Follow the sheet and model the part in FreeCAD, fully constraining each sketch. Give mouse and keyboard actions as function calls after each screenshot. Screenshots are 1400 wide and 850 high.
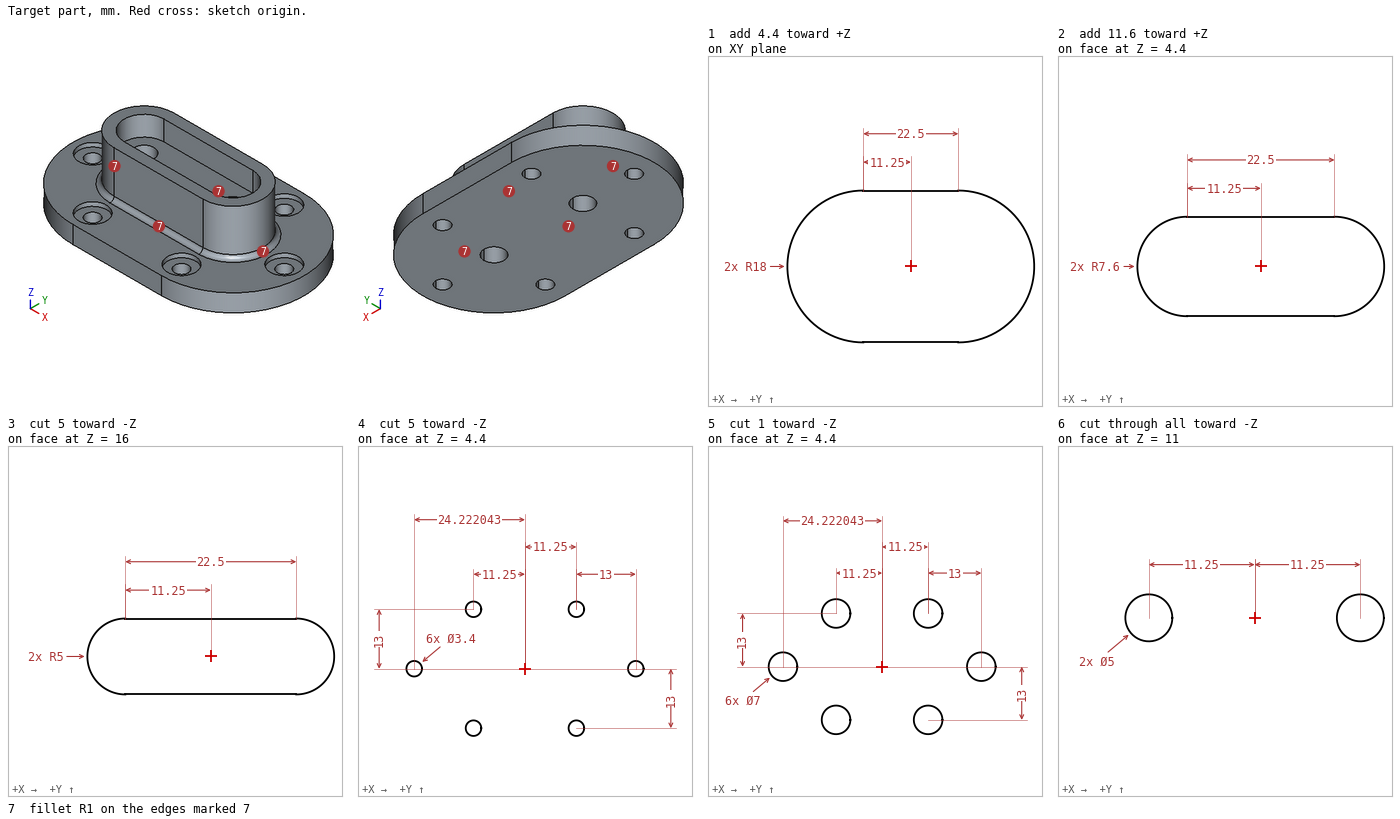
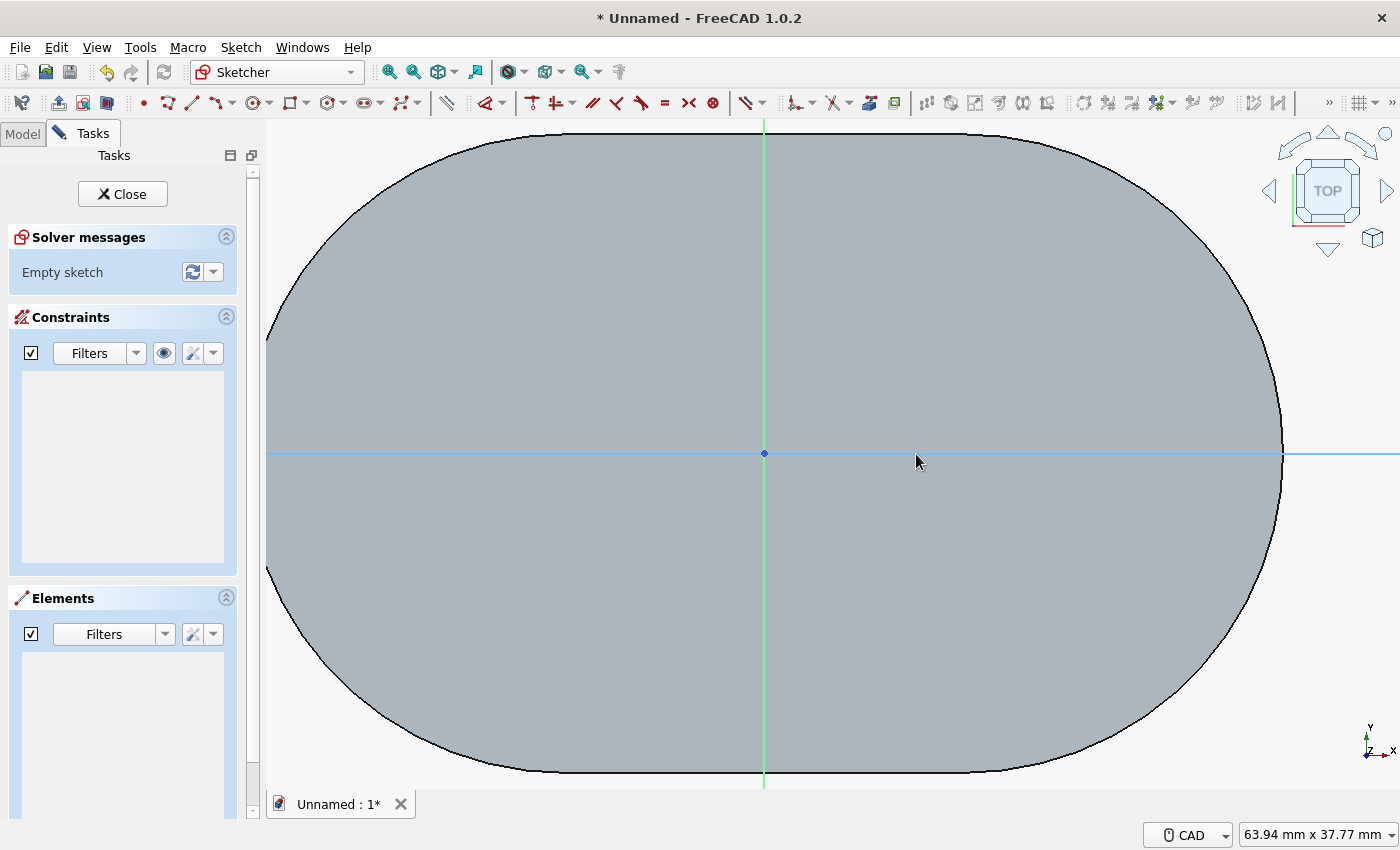
click(364, 104)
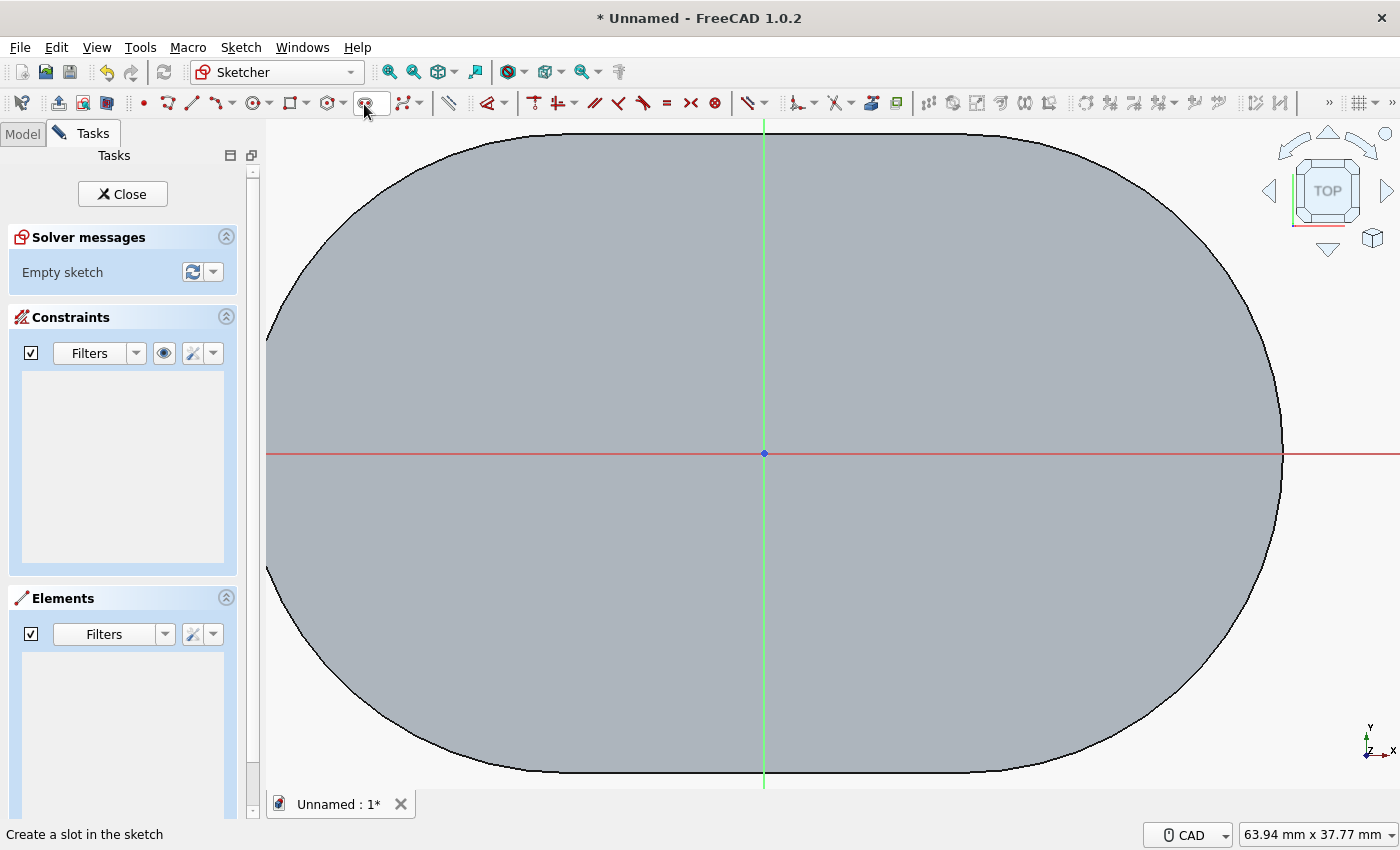
click(565, 454)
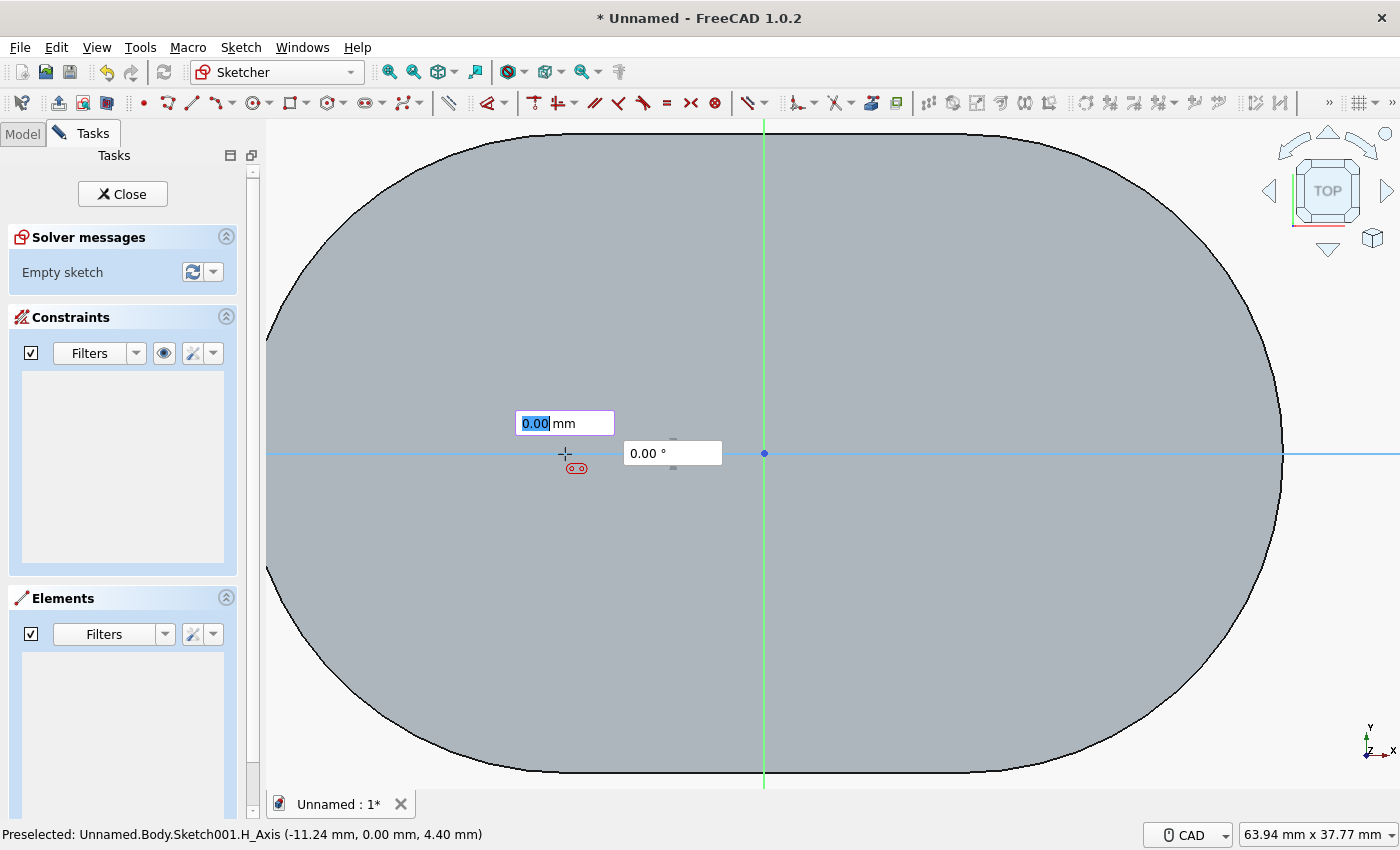
click(964, 445)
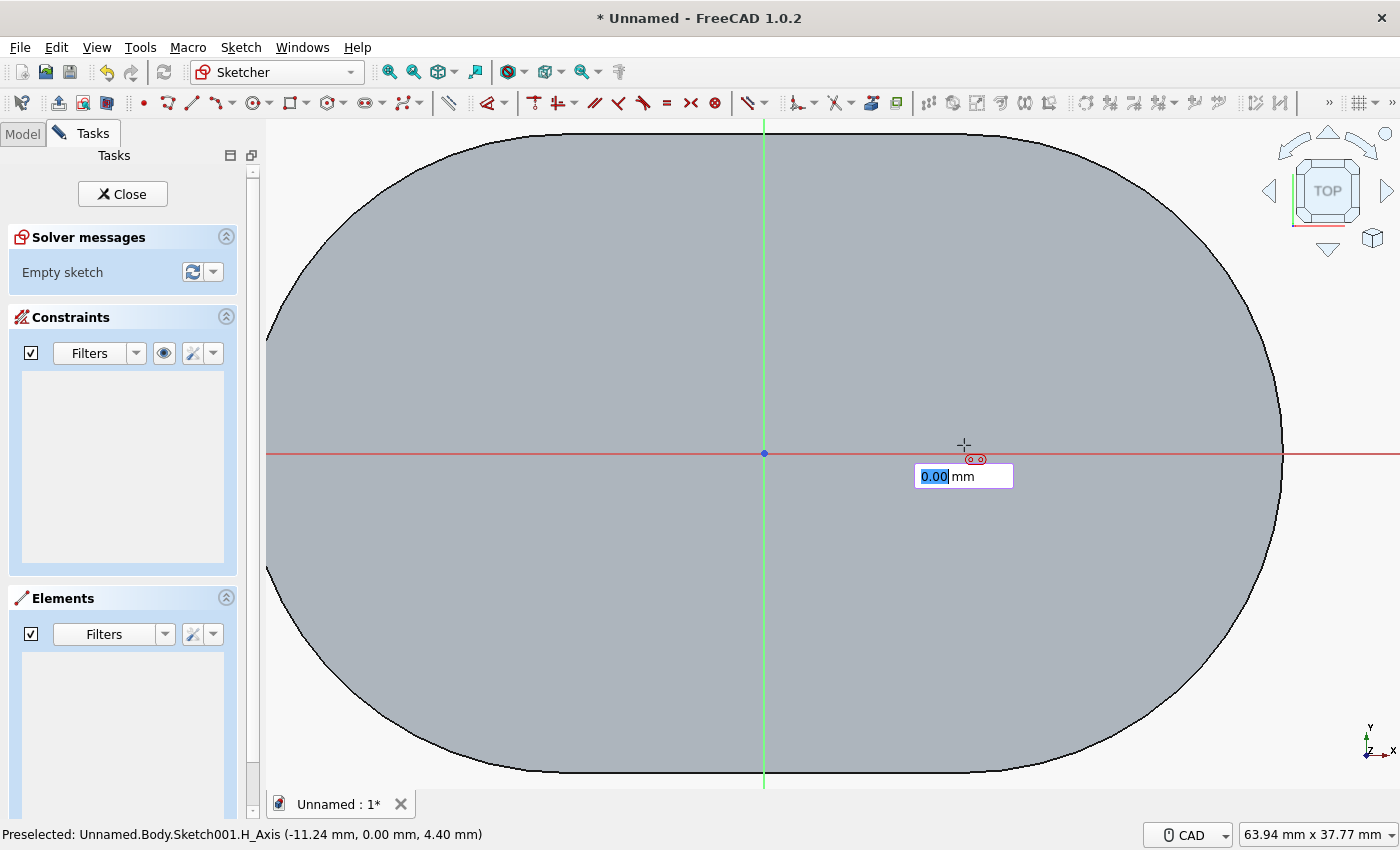
click(824, 319)
key(Escape)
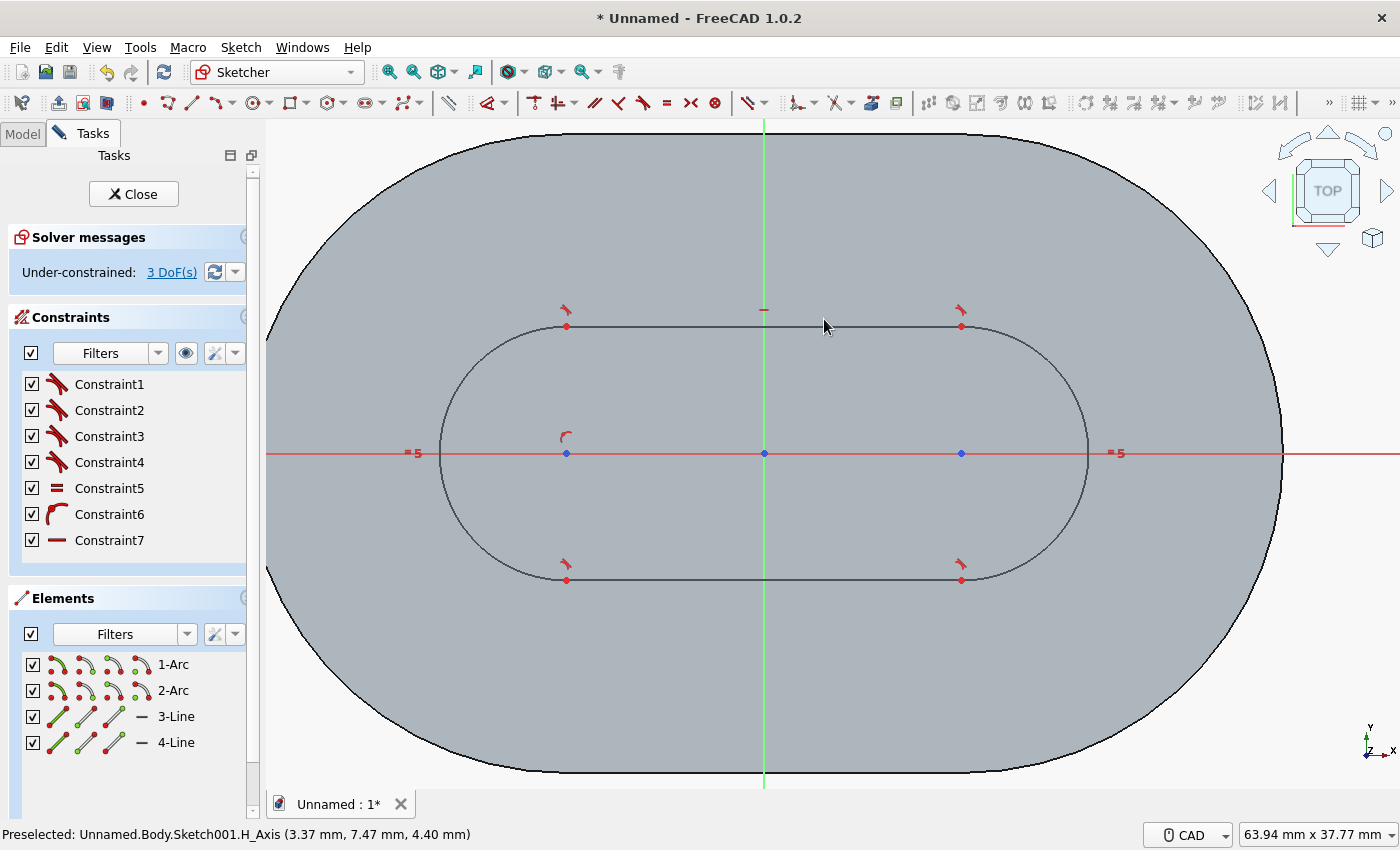
click(488, 104)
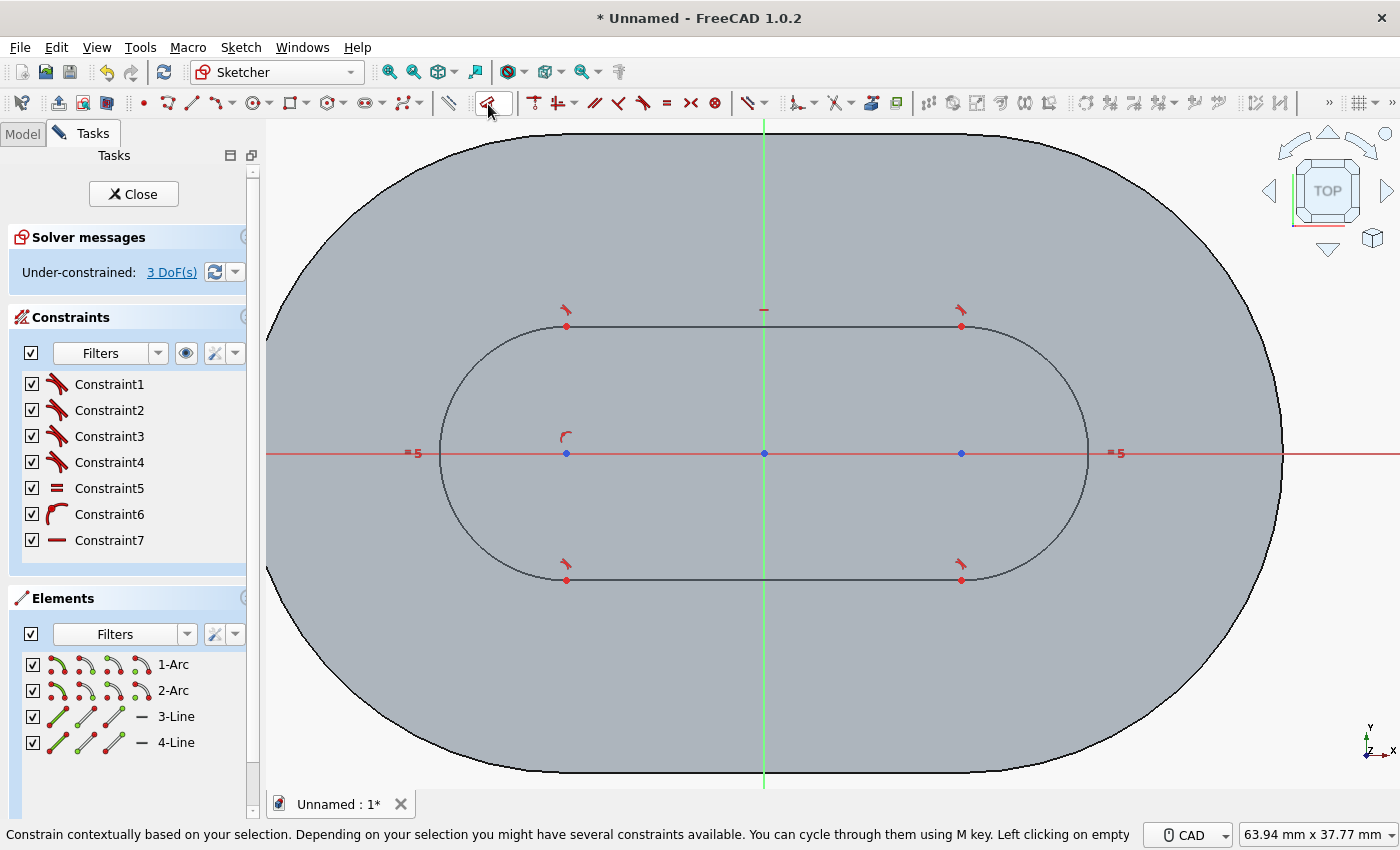
click(464, 379)
click(438, 360)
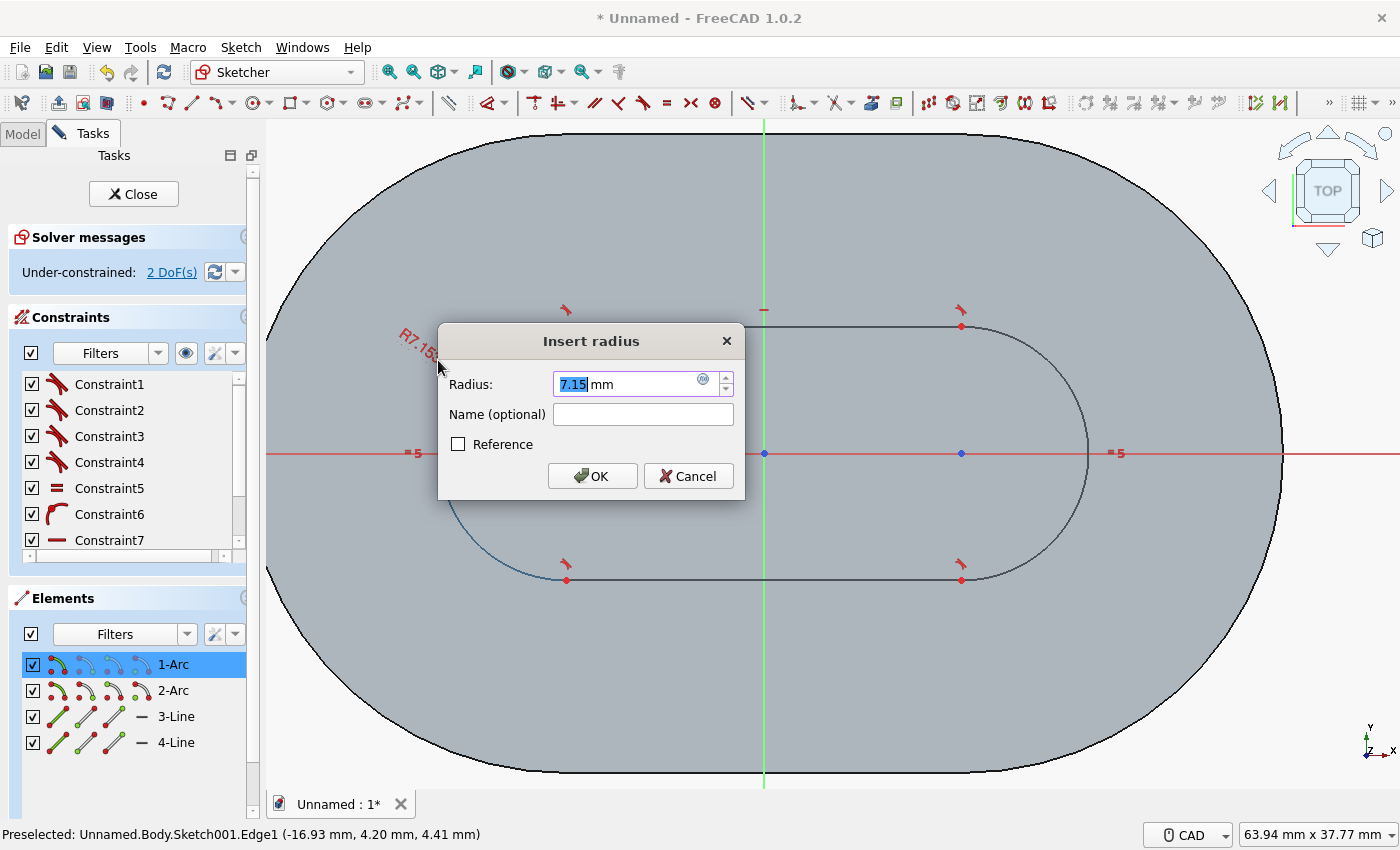
text(7.6)
key(Return)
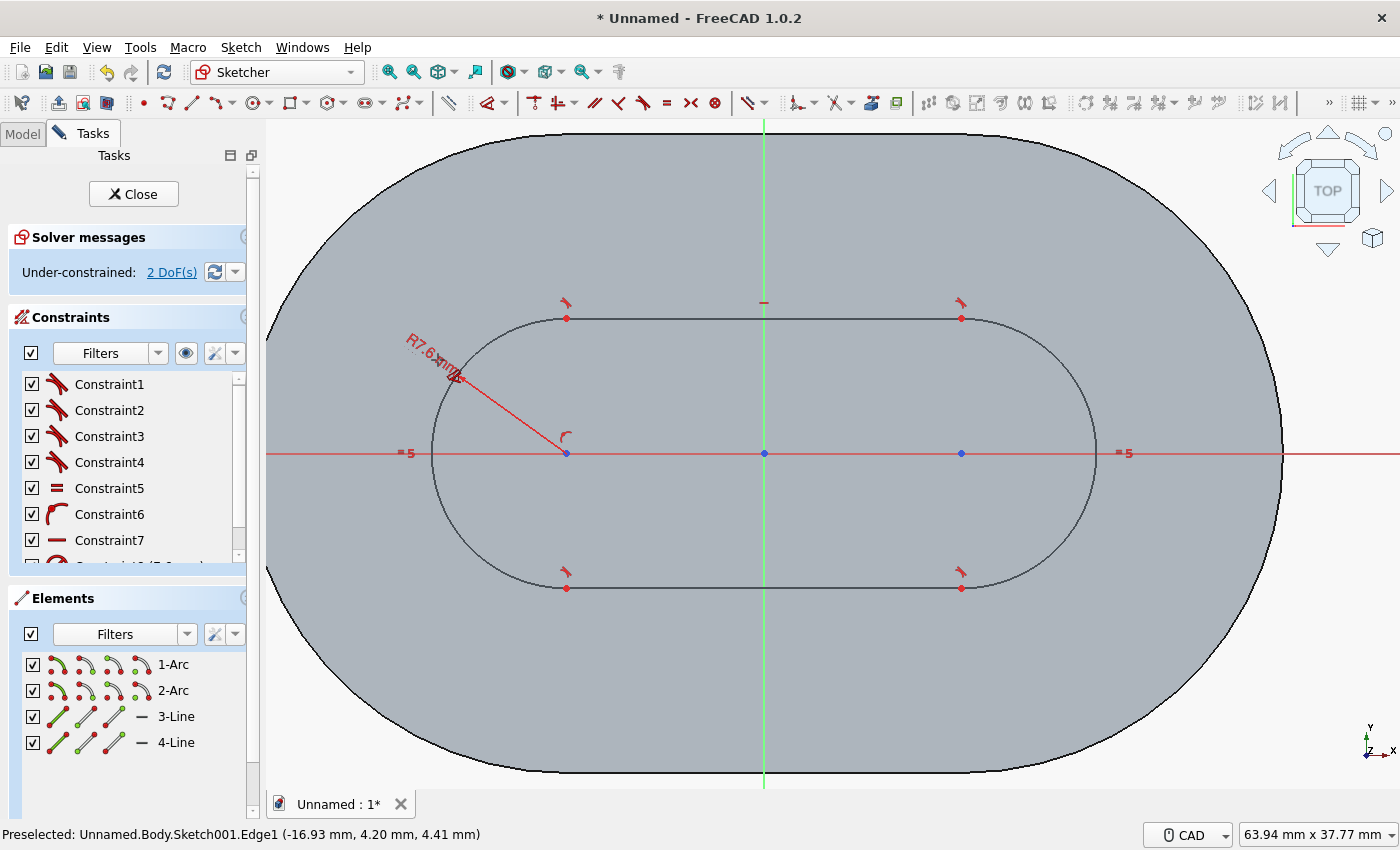
click(685, 319)
click(673, 285)